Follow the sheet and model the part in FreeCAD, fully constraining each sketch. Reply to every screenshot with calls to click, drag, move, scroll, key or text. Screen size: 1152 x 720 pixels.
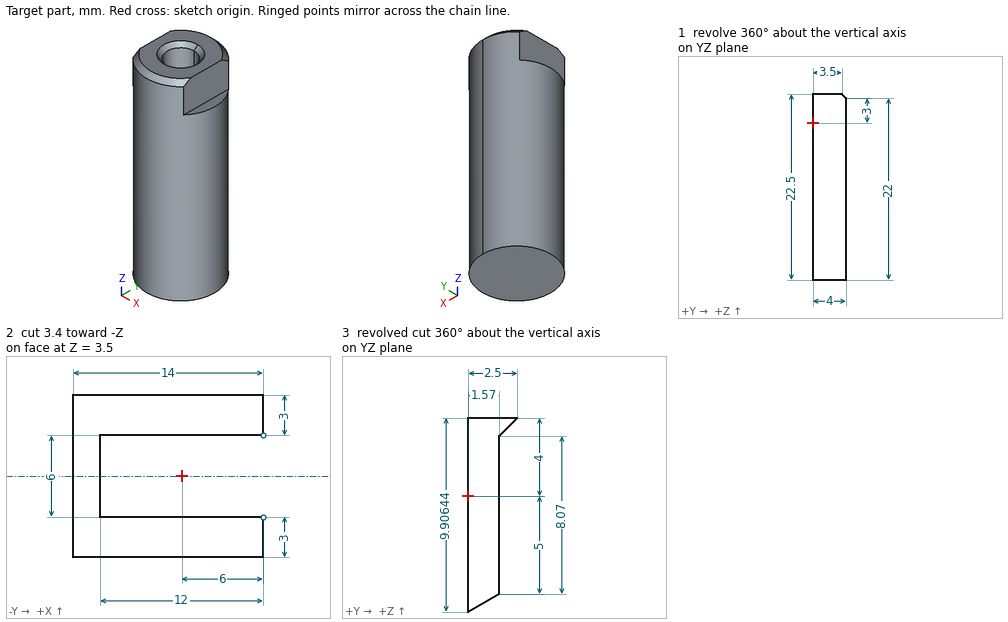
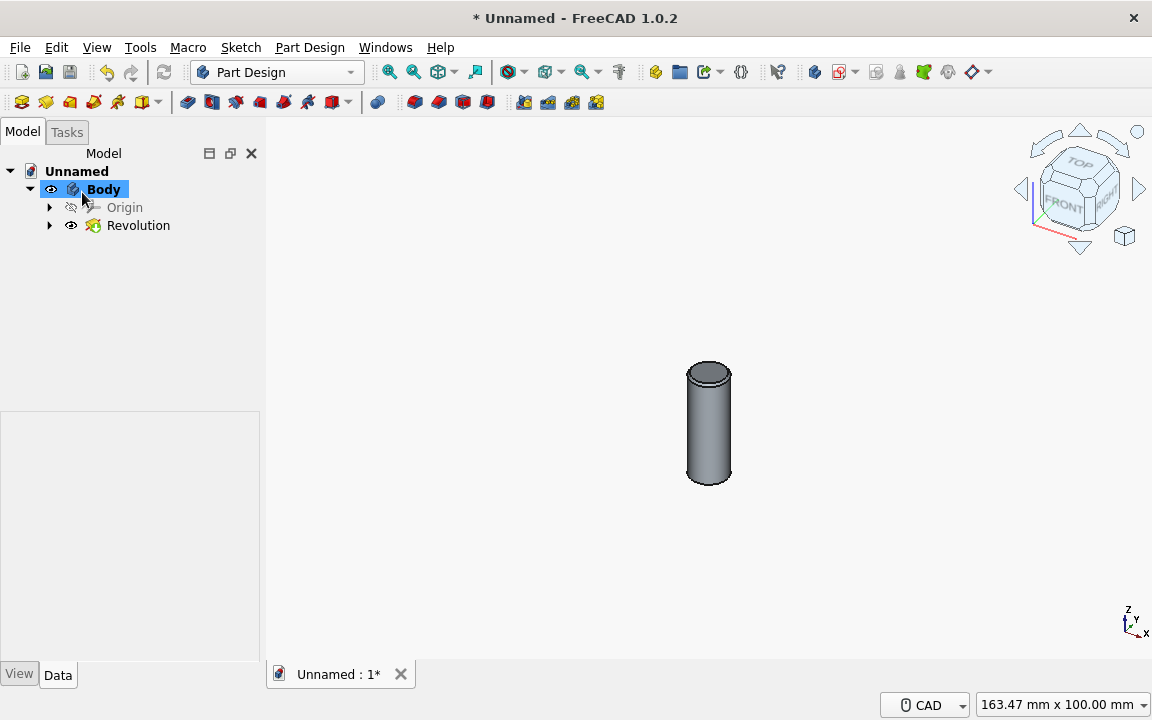
click(390, 72)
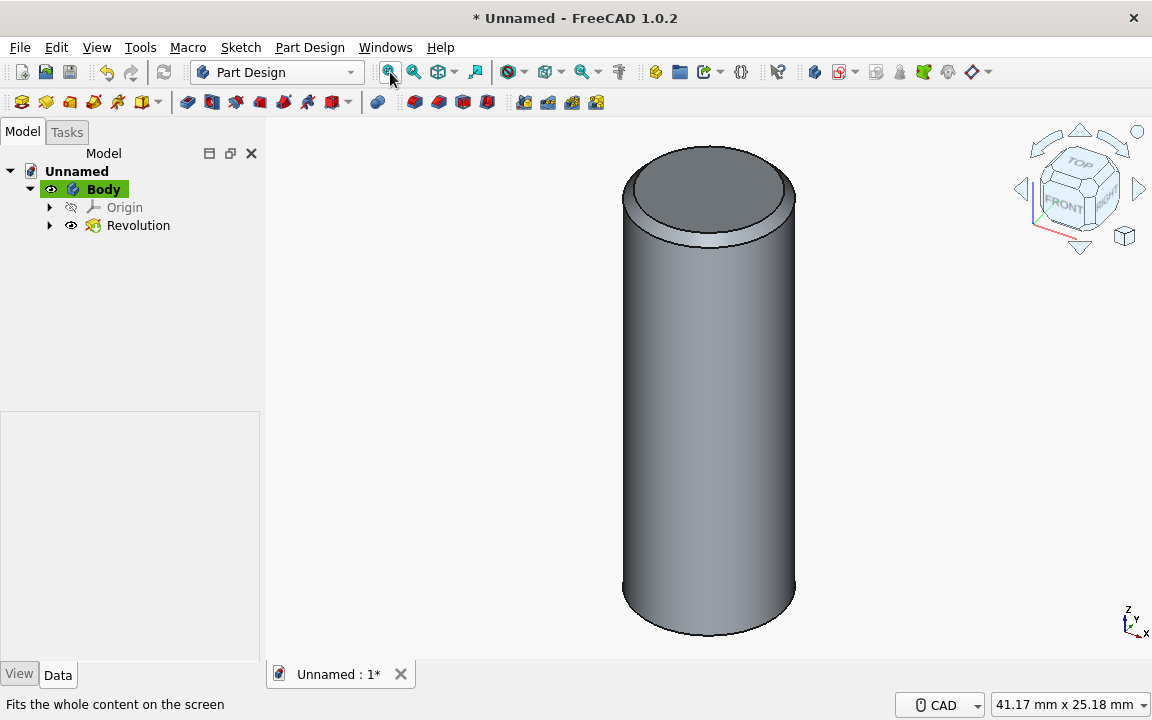
click(709, 189)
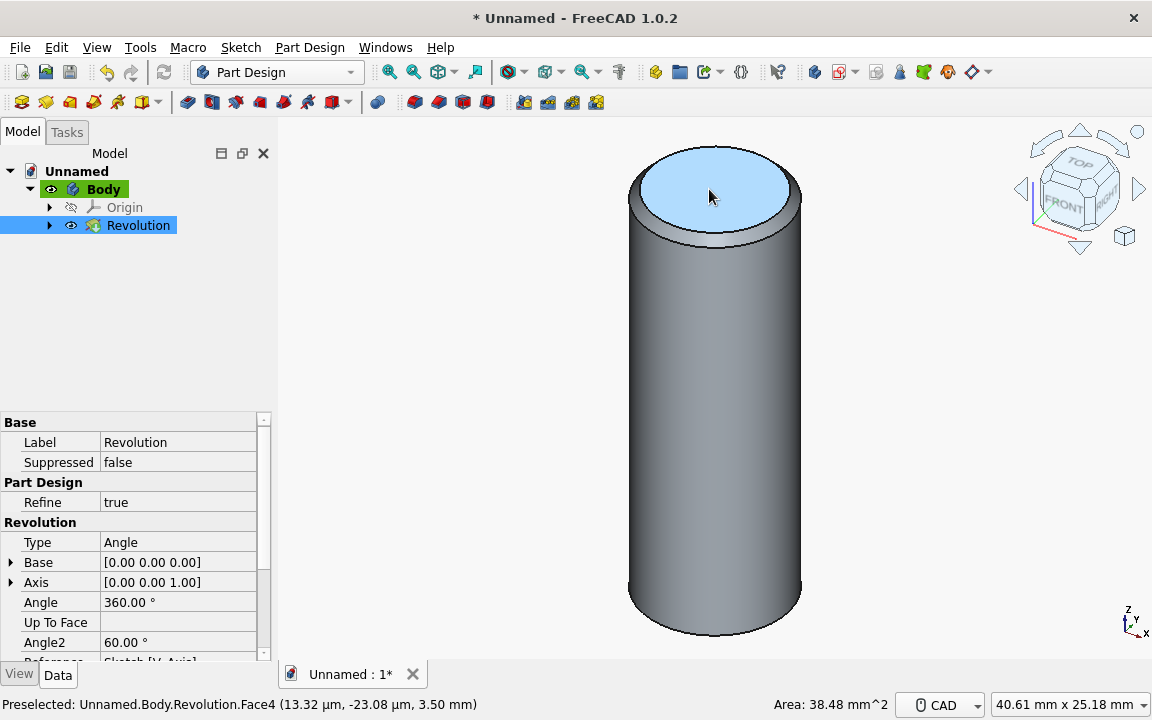
click(840, 72)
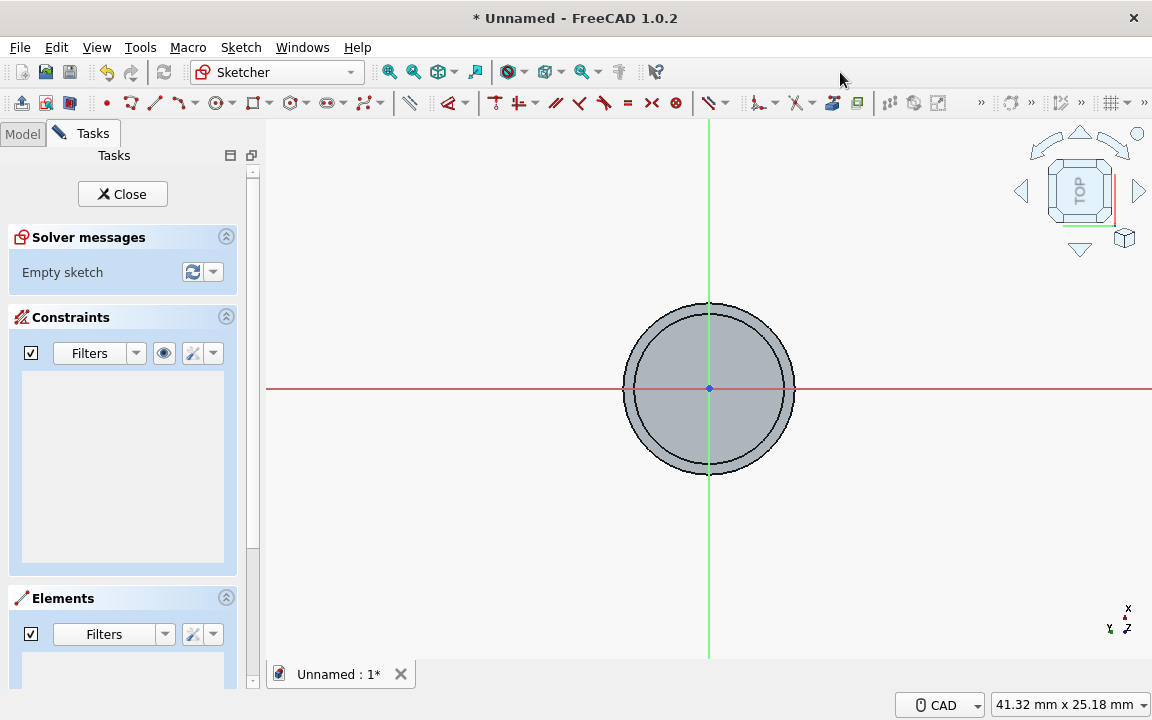
click(132, 104)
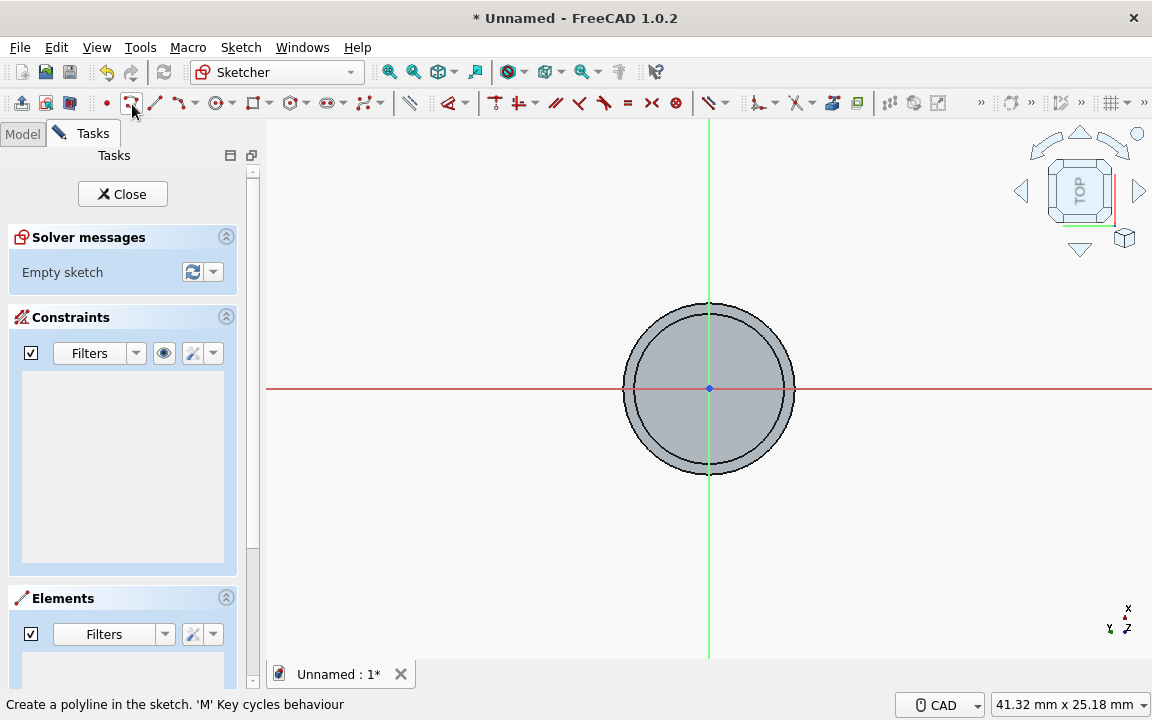
click(838, 453)
click(580, 453)
click(580, 325)
click(838, 325)
click(838, 260)
click(537, 260)
click(537, 518)
click(838, 518)
click(838, 454)
key(Escape)
key(Escape)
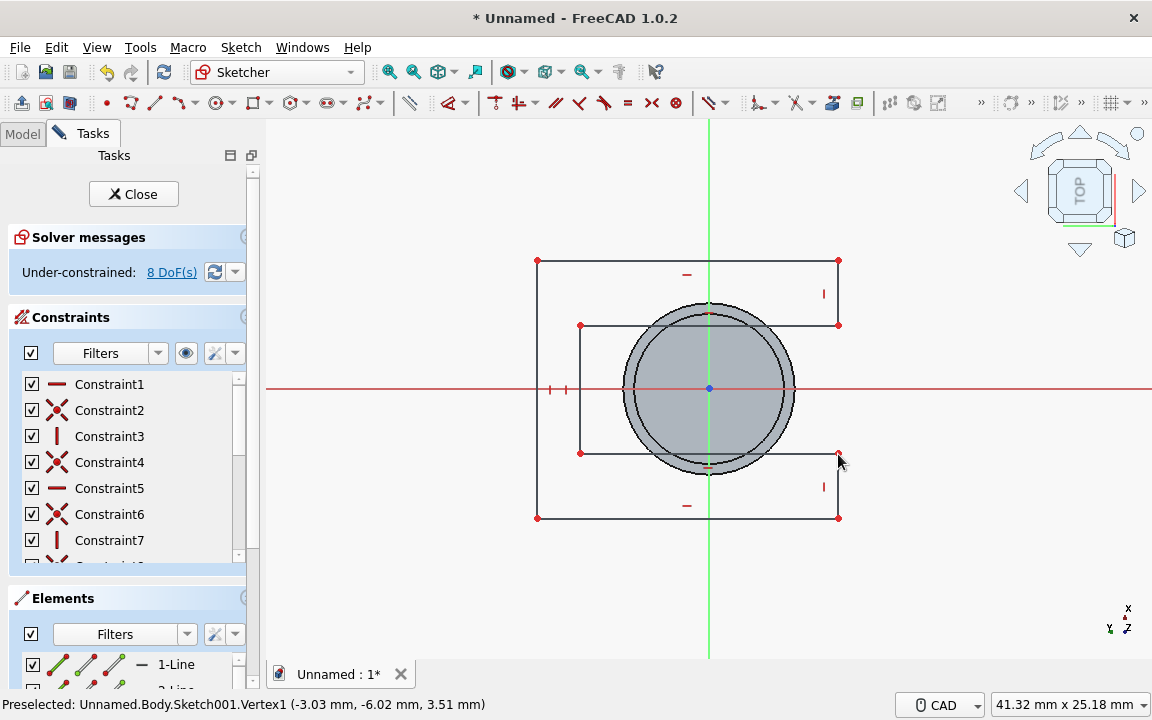
click(838, 454)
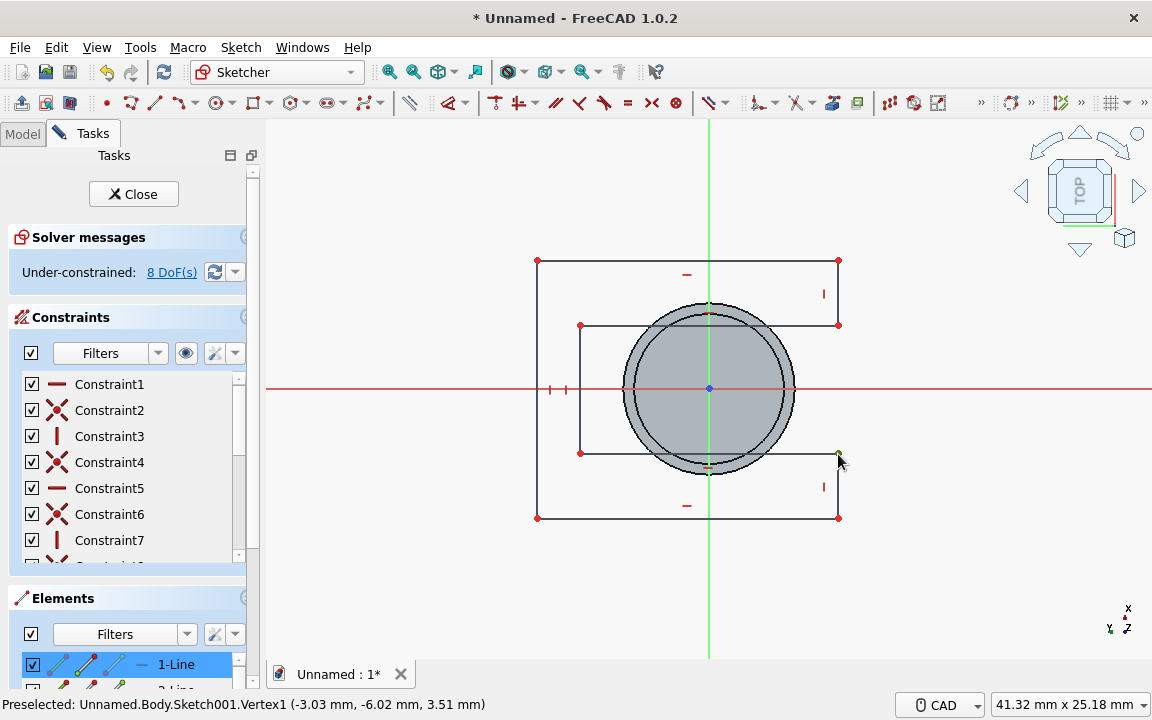
click(838, 326)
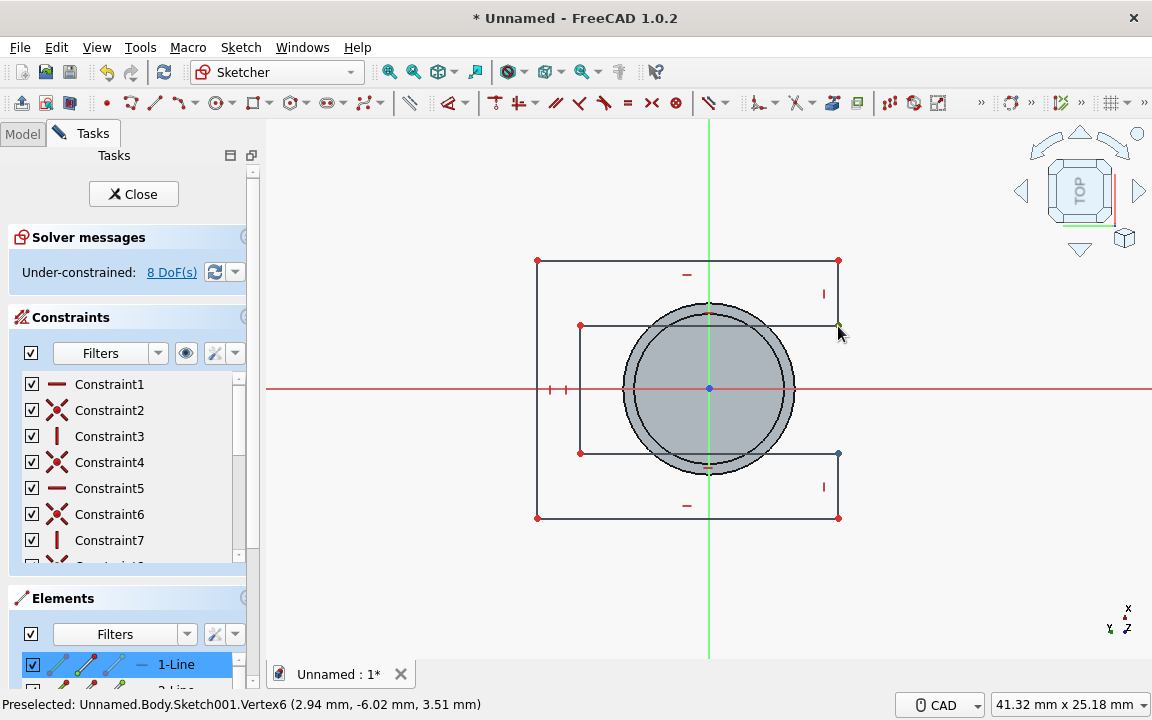
click(344, 389)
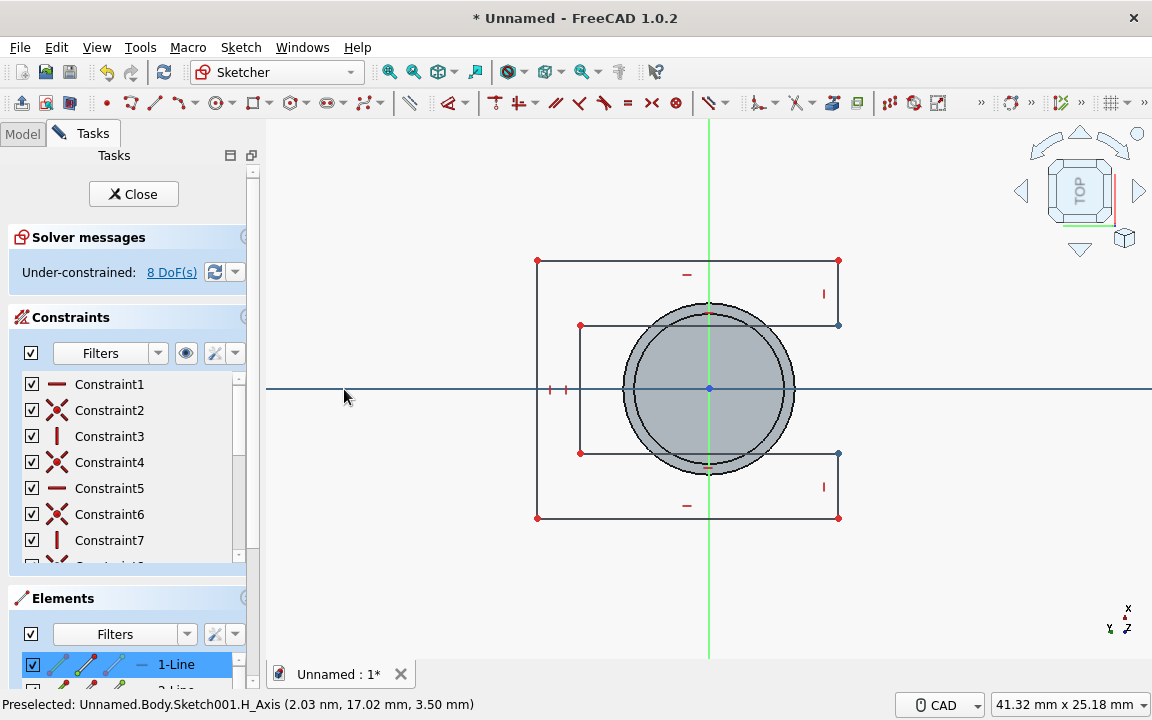
click(652, 104)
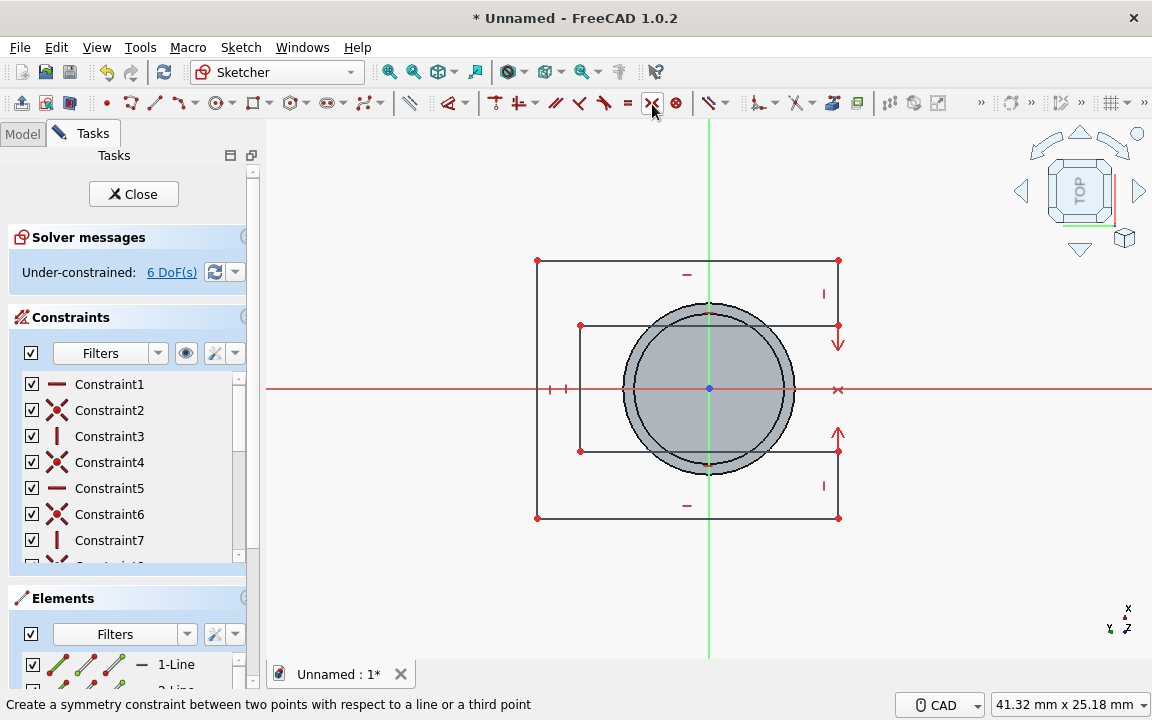
click(448, 104)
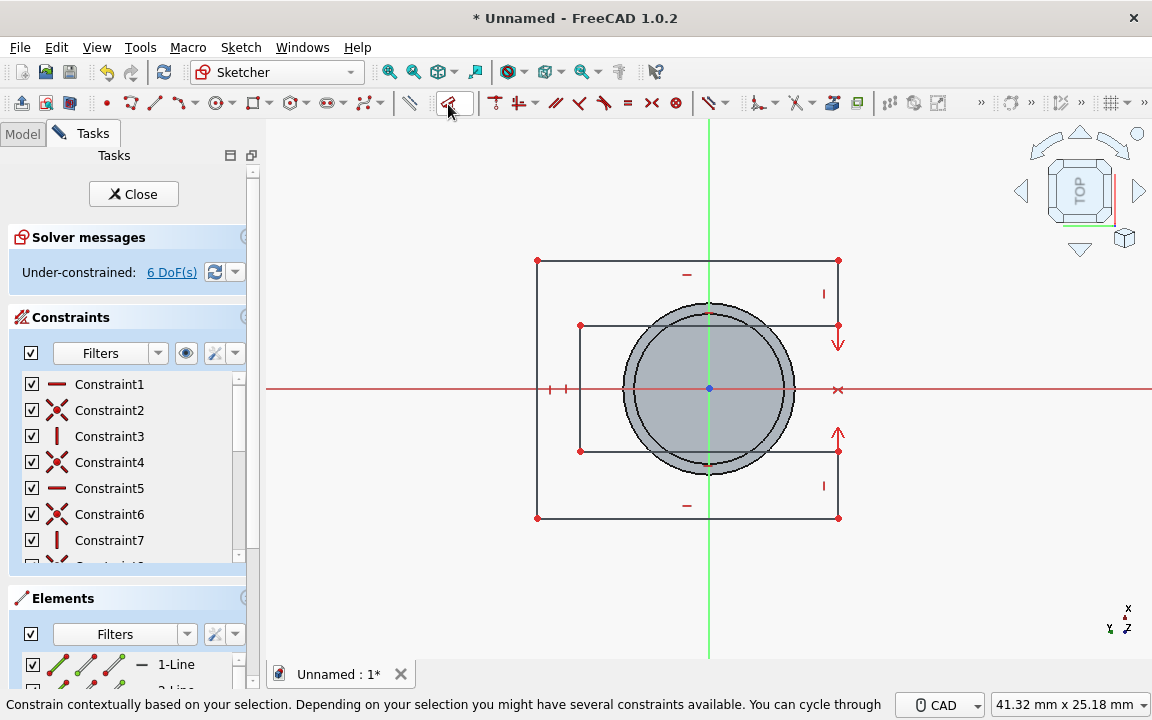
click(580, 414)
click(614, 360)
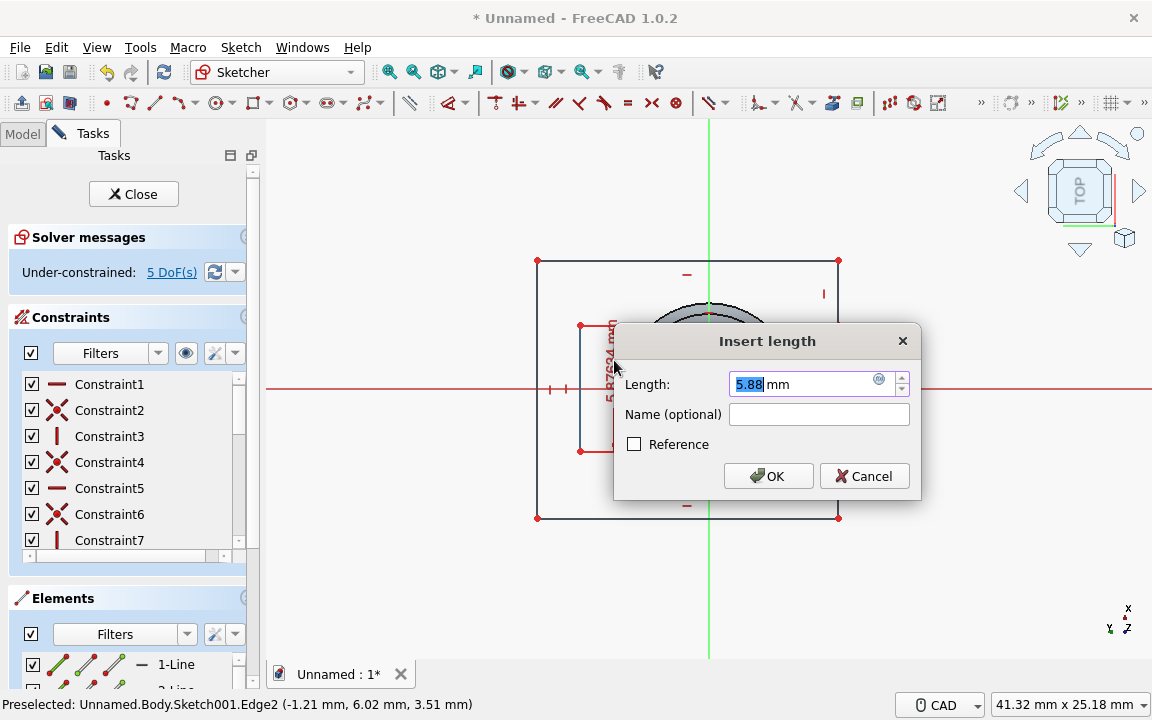
text(6)
key(Return)